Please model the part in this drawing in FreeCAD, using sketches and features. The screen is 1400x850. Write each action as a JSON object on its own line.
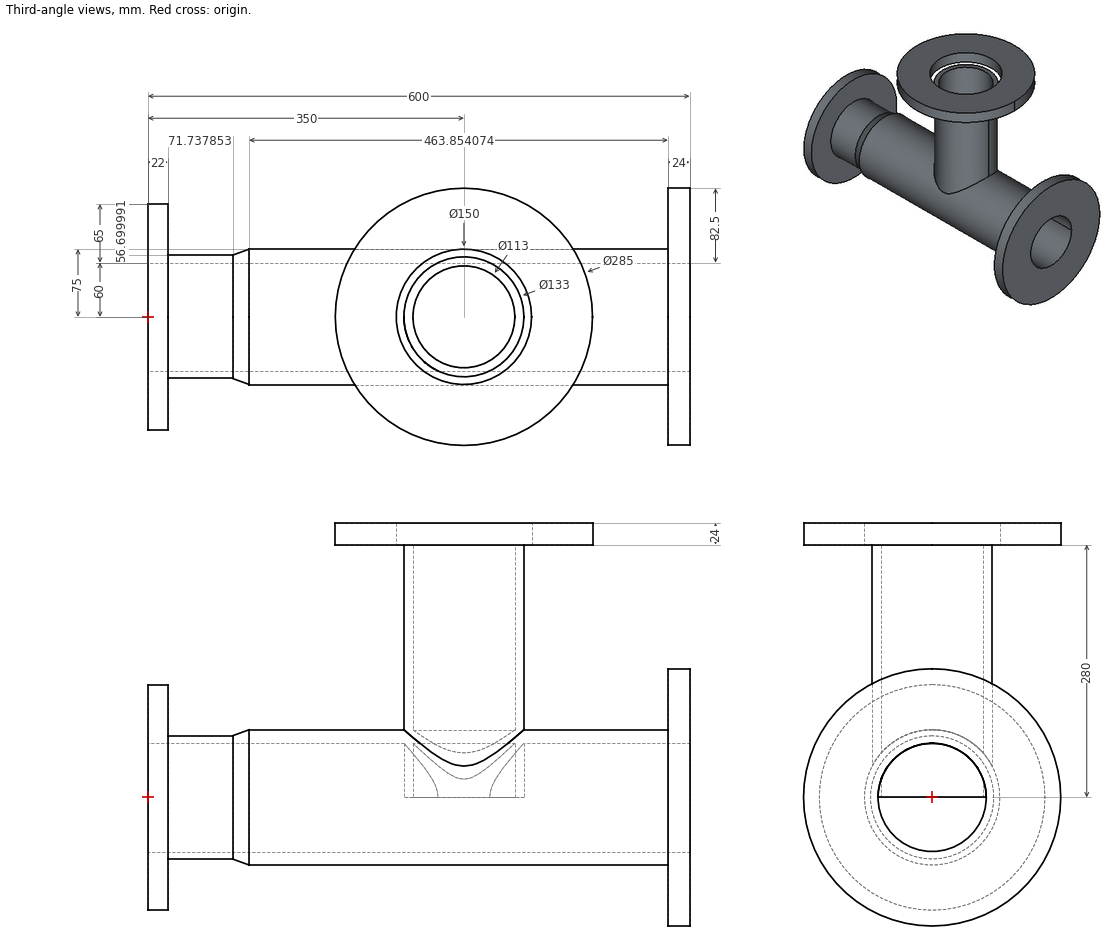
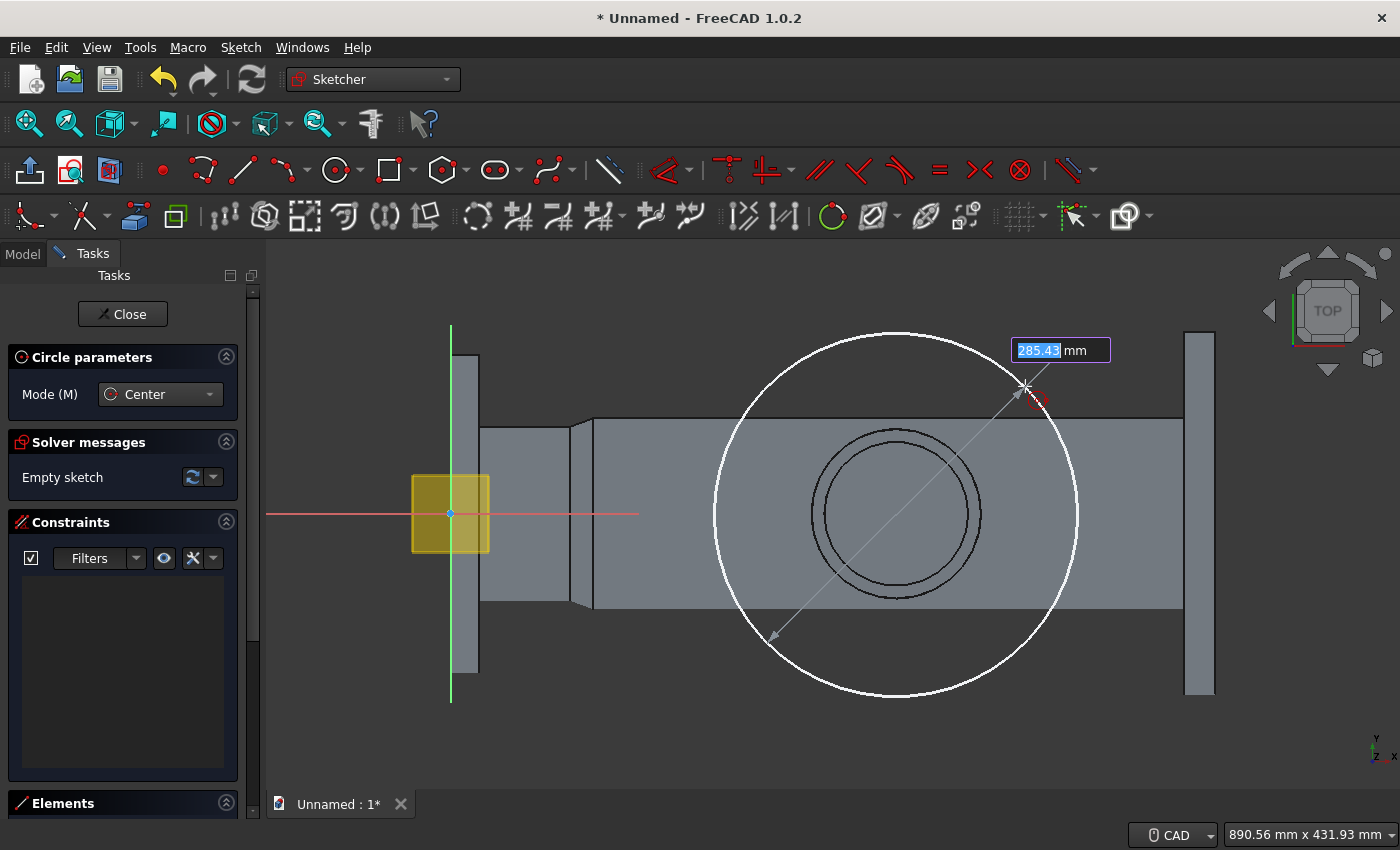
{"action": "type", "text": "285"}
{"action": "key", "text": "Return"}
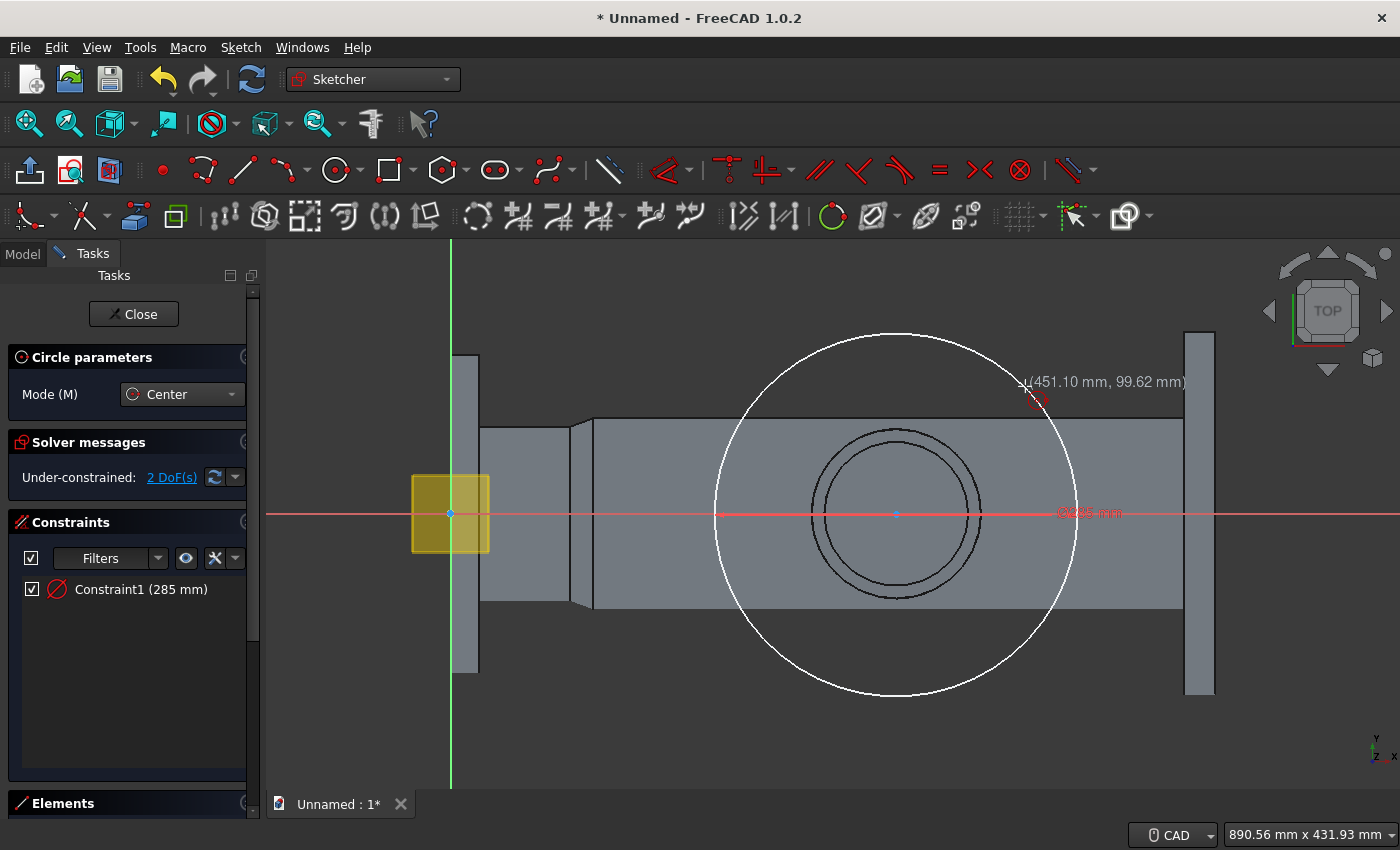
{"action": "left_click", "coordinate": [896, 515]}
{"action": "mouse_move", "coordinate": [964, 446]}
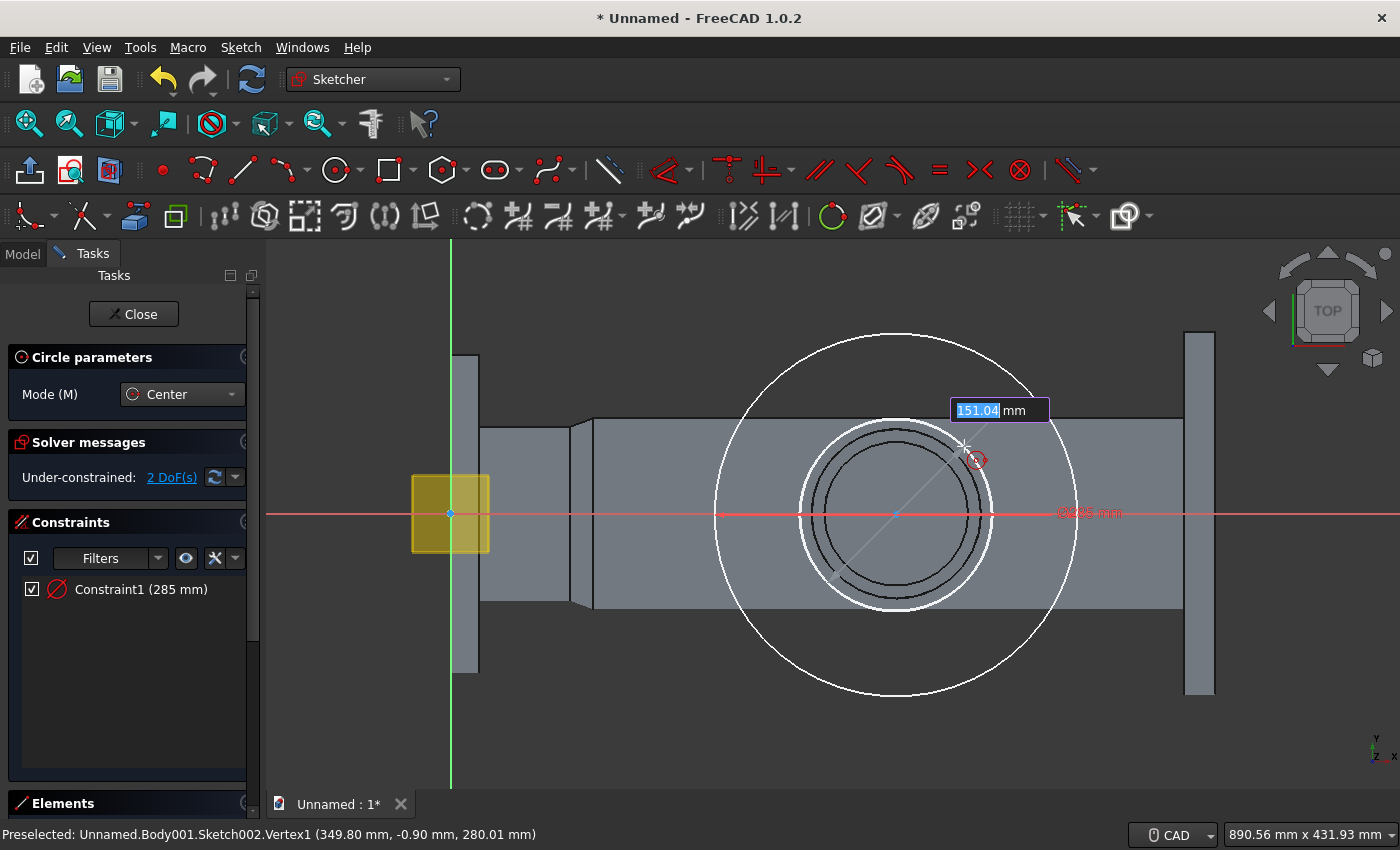
{"action": "type", "text": "150"}
{"action": "key", "text": "Return"}
{"action": "key", "text": "Escape"}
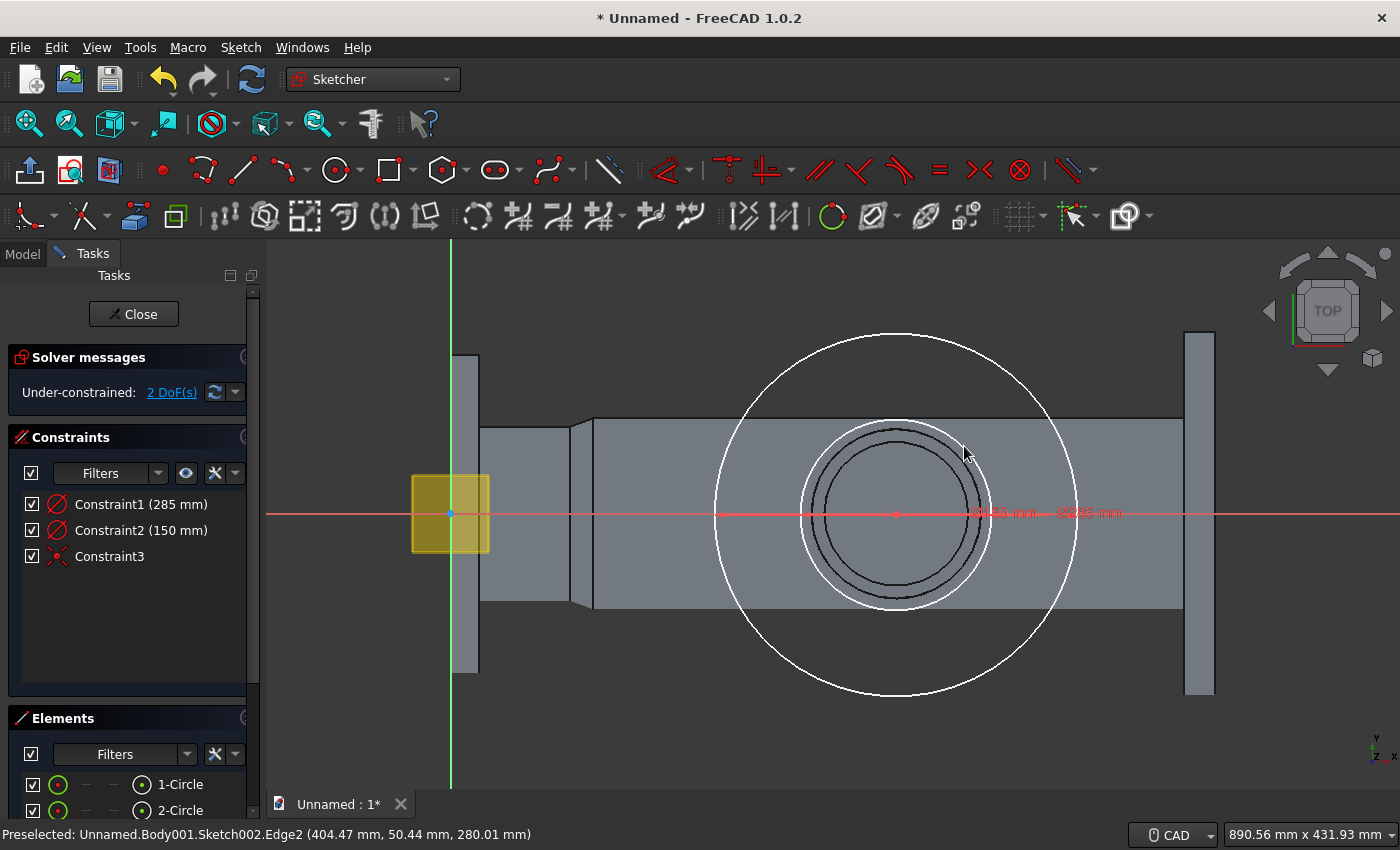
{"action": "left_click", "coordinate": [896, 515]}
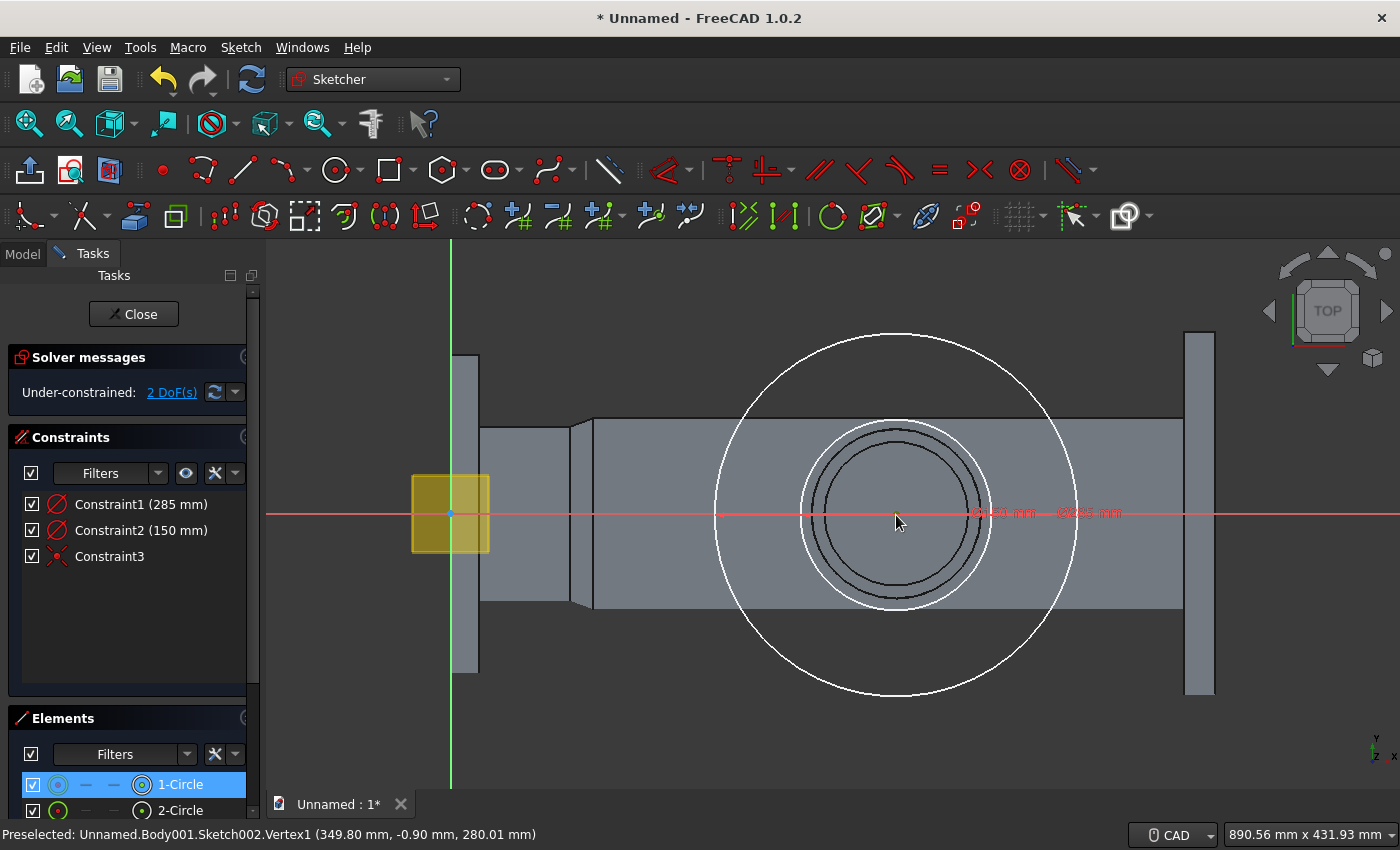
{"action": "left_click", "coordinate": [361, 514]}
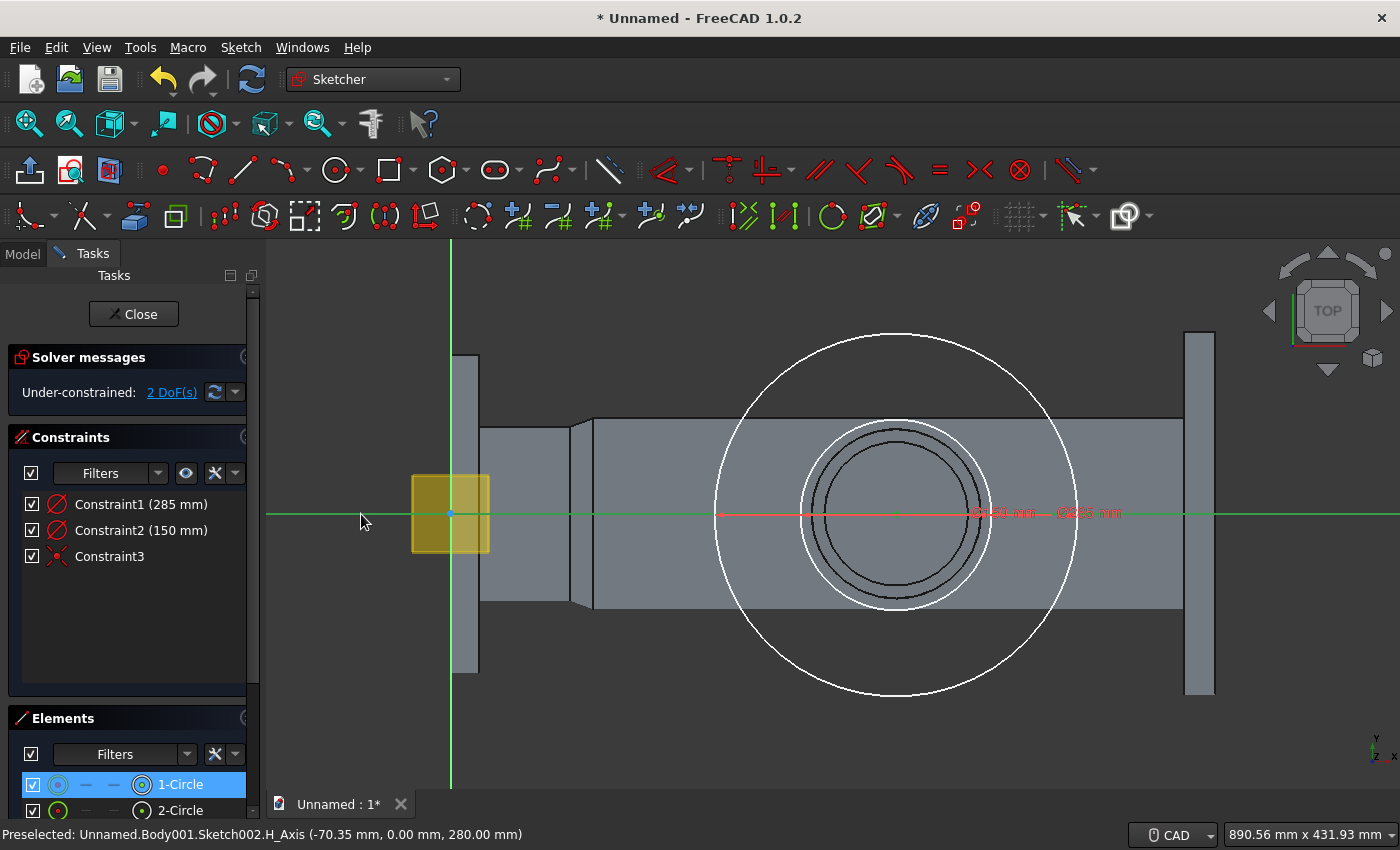
{"action": "key", "text": "c"}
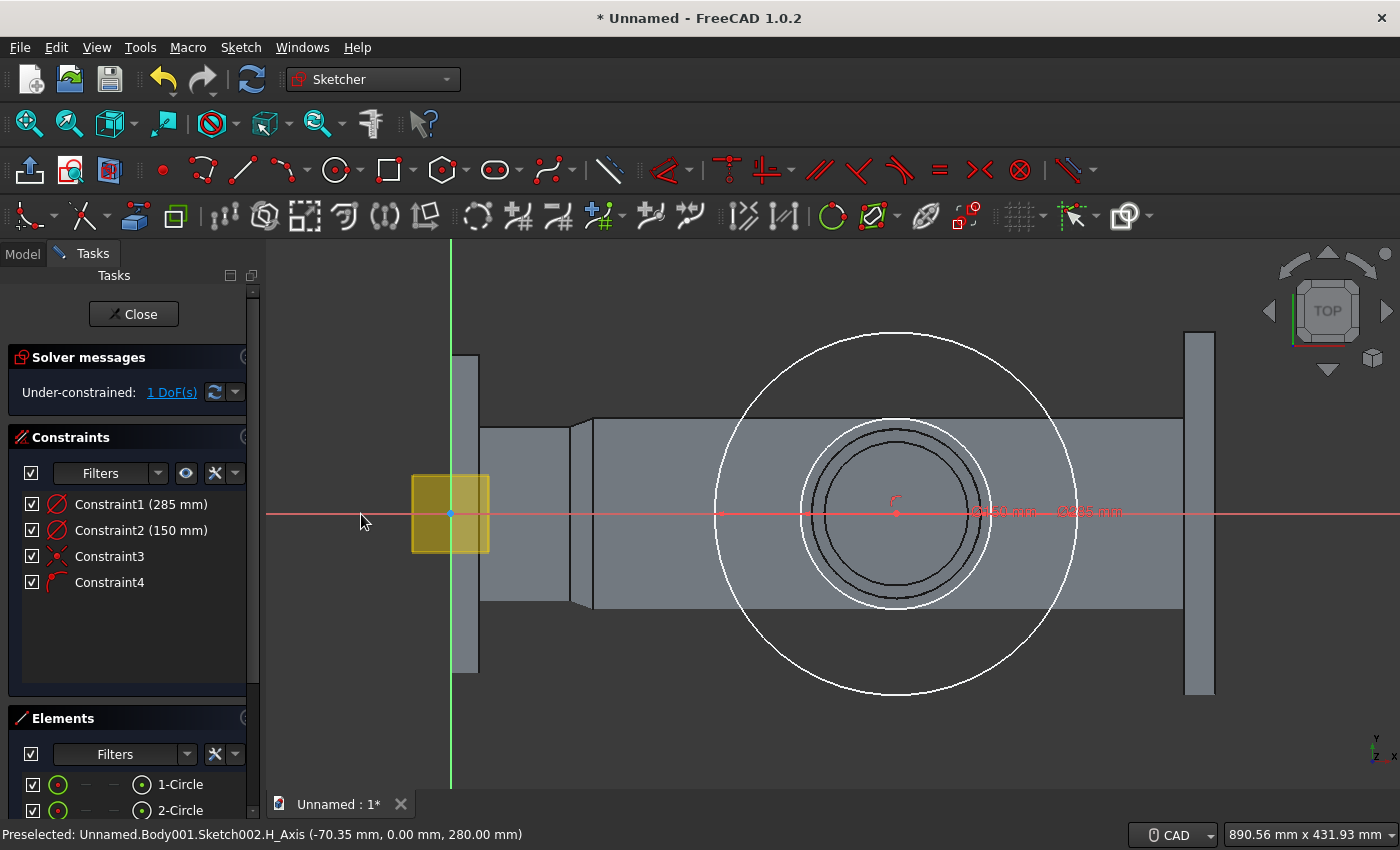
{"action": "key", "text": "d"}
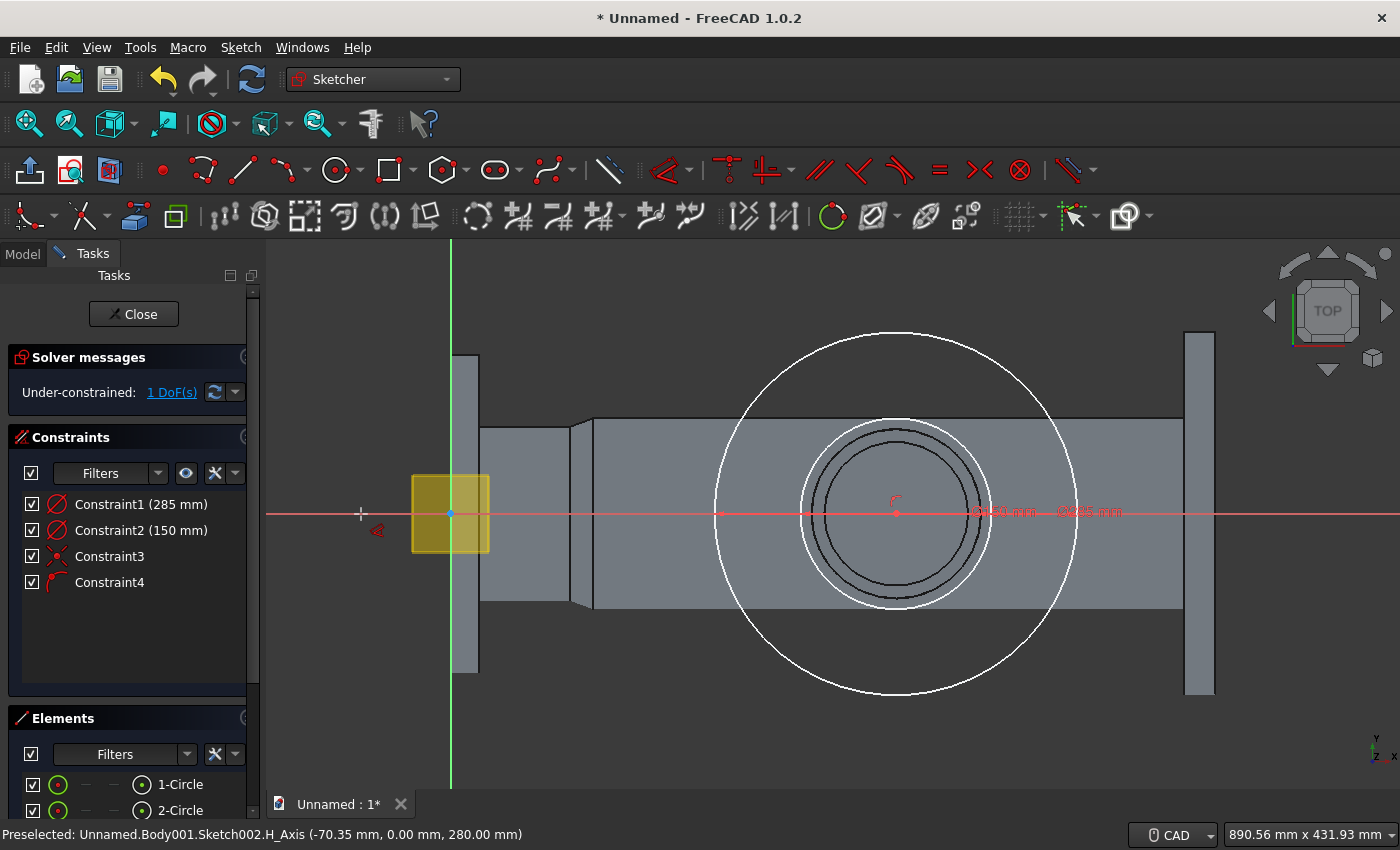
{"action": "left_click", "coordinate": [896, 514]}
{"action": "left_click", "coordinate": [673, 548]}